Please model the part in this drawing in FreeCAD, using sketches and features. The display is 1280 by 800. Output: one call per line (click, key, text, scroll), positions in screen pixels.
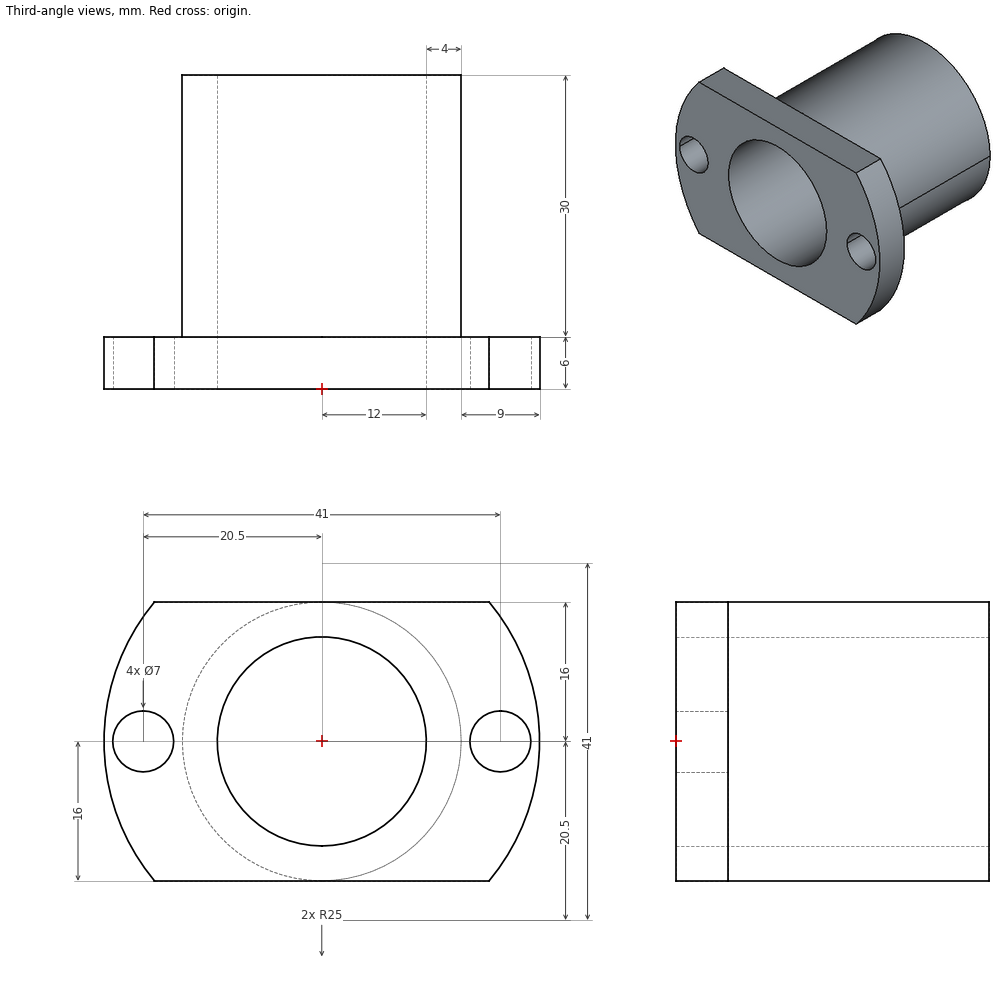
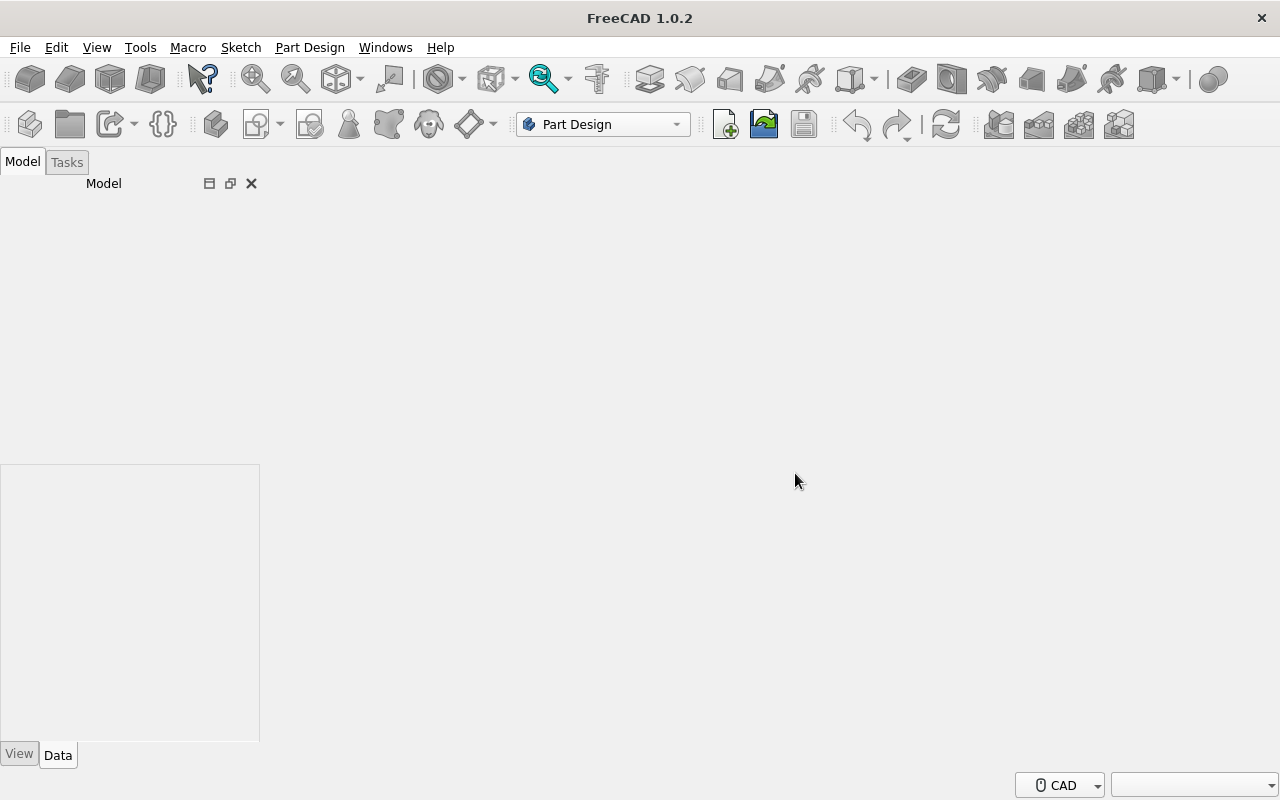
click(724, 124)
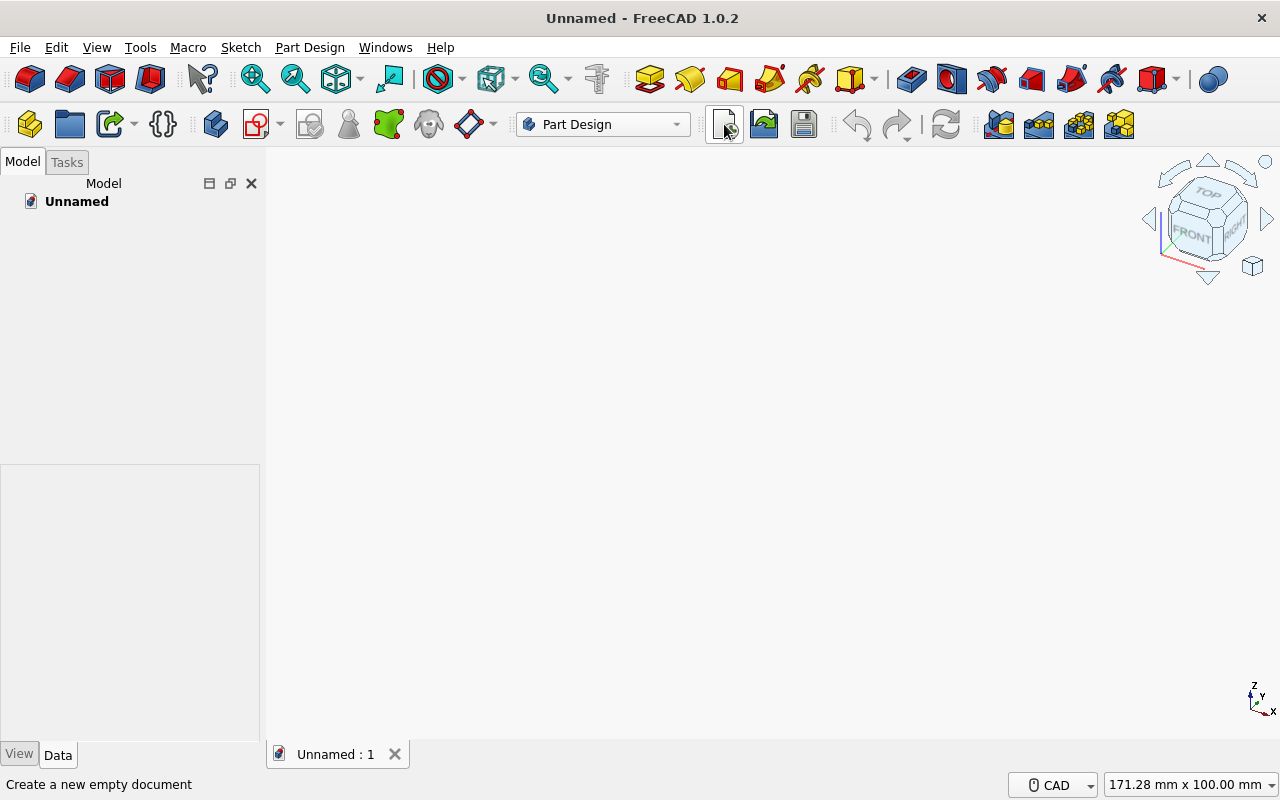
click(256, 124)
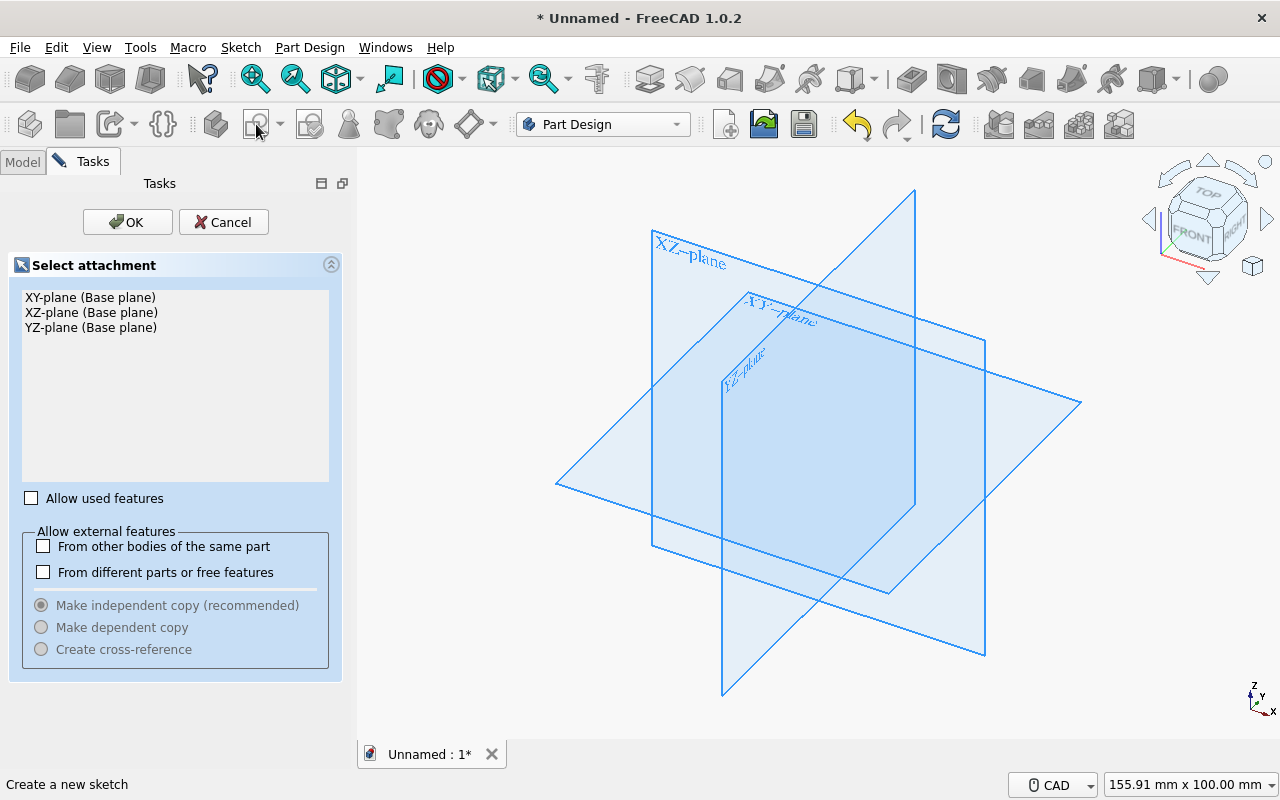
click(82, 298)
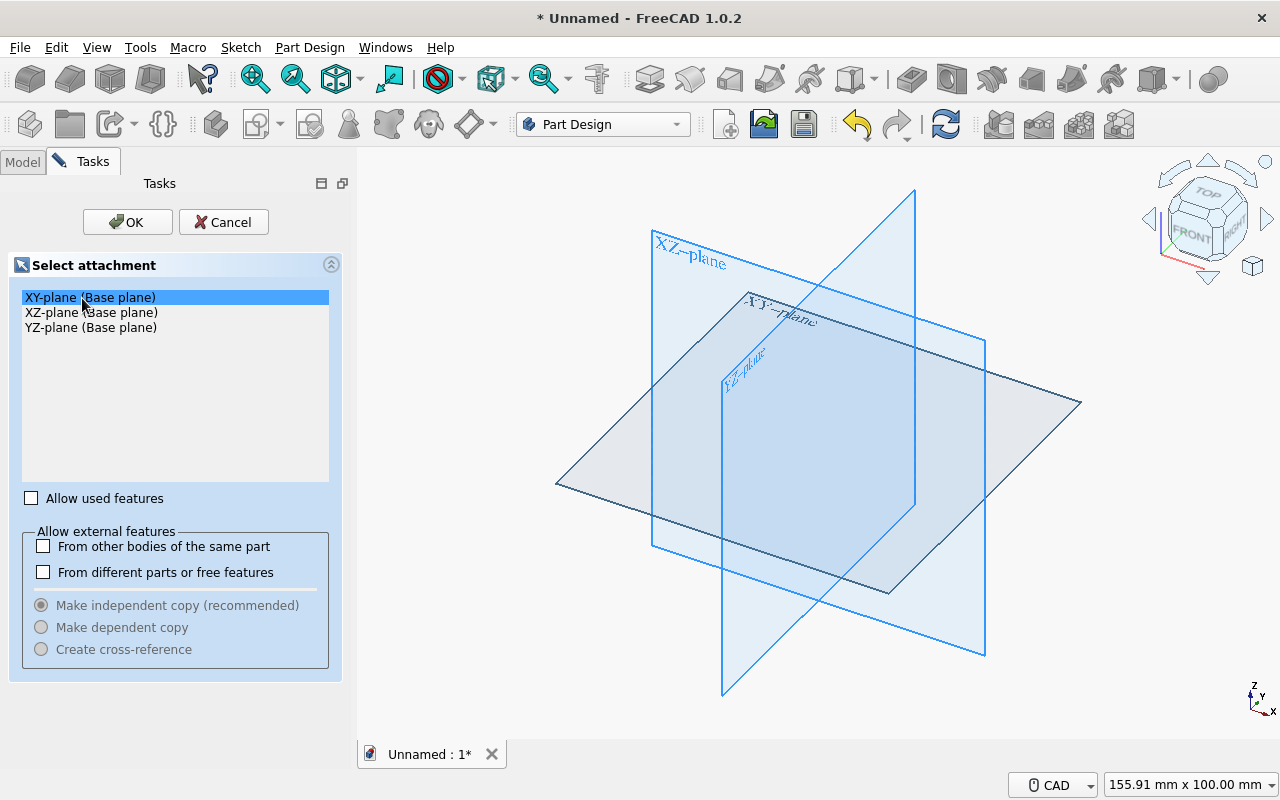
click(128, 222)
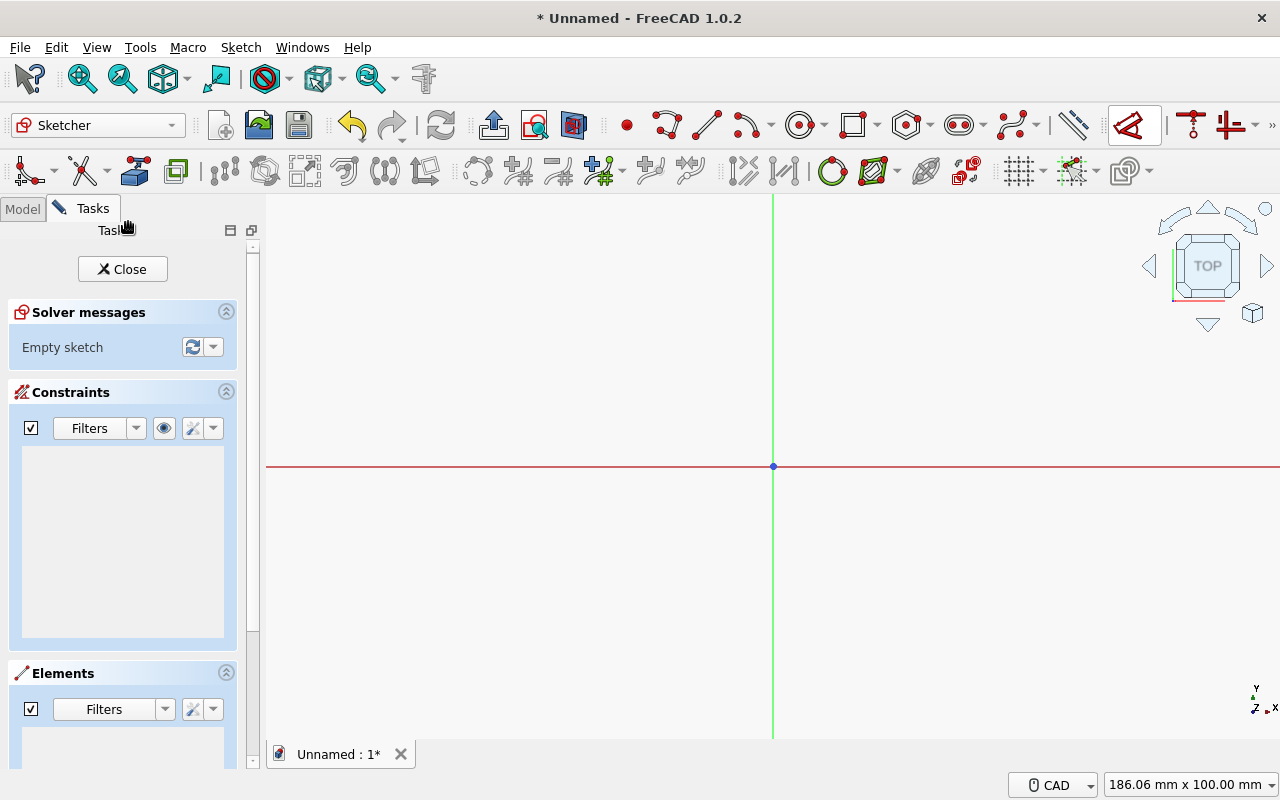
scroll(1007, 249, up, 3)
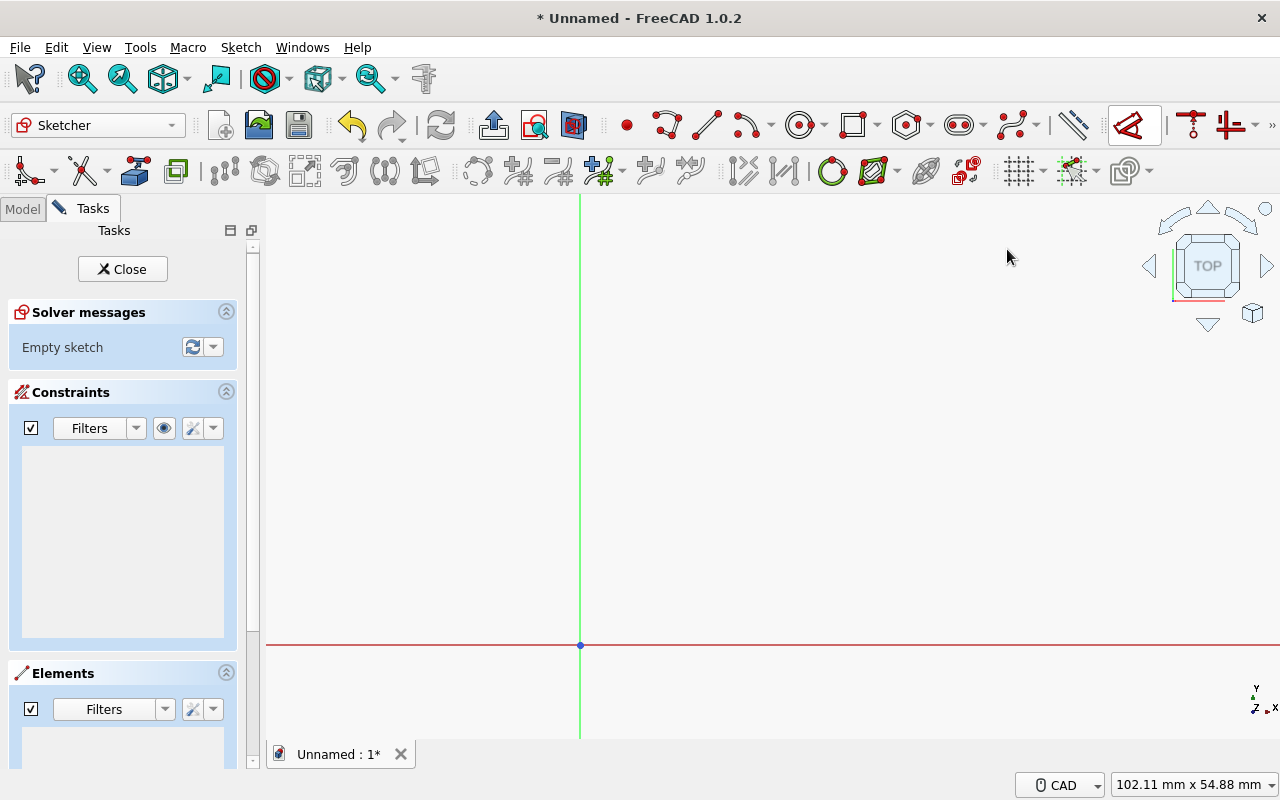
click(668, 126)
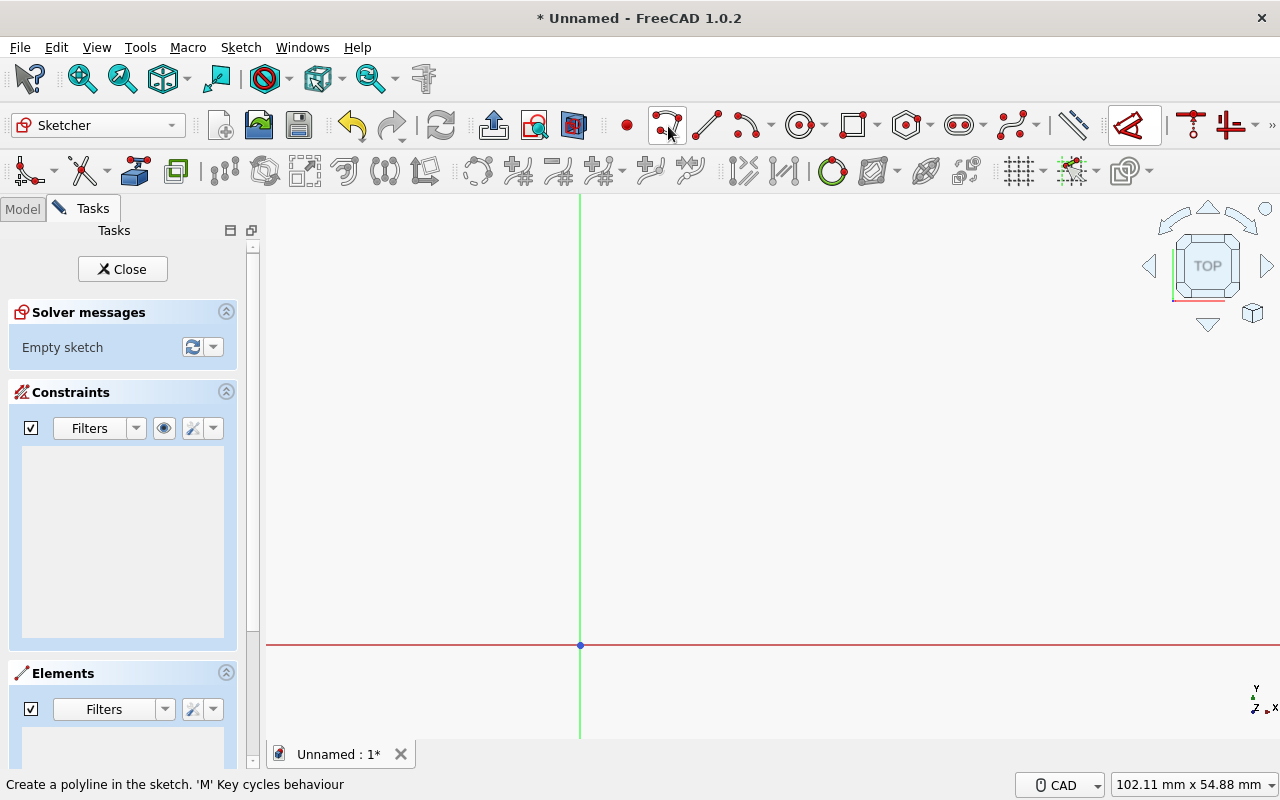
click(699, 645)
click(828, 636)
click(828, 586)
click(739, 586)
click(739, 288)
click(699, 288)
click(699, 645)
key(Escape)
key(Escape)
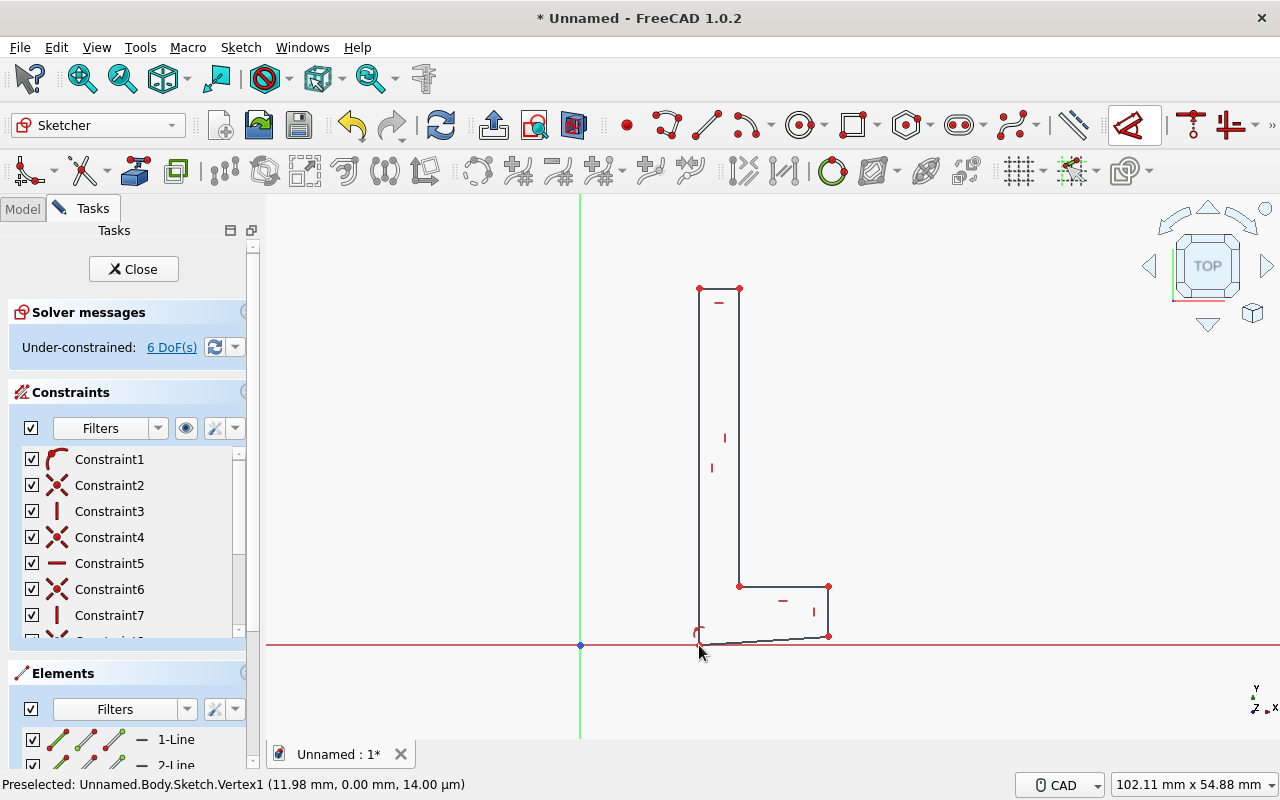
click(738, 643)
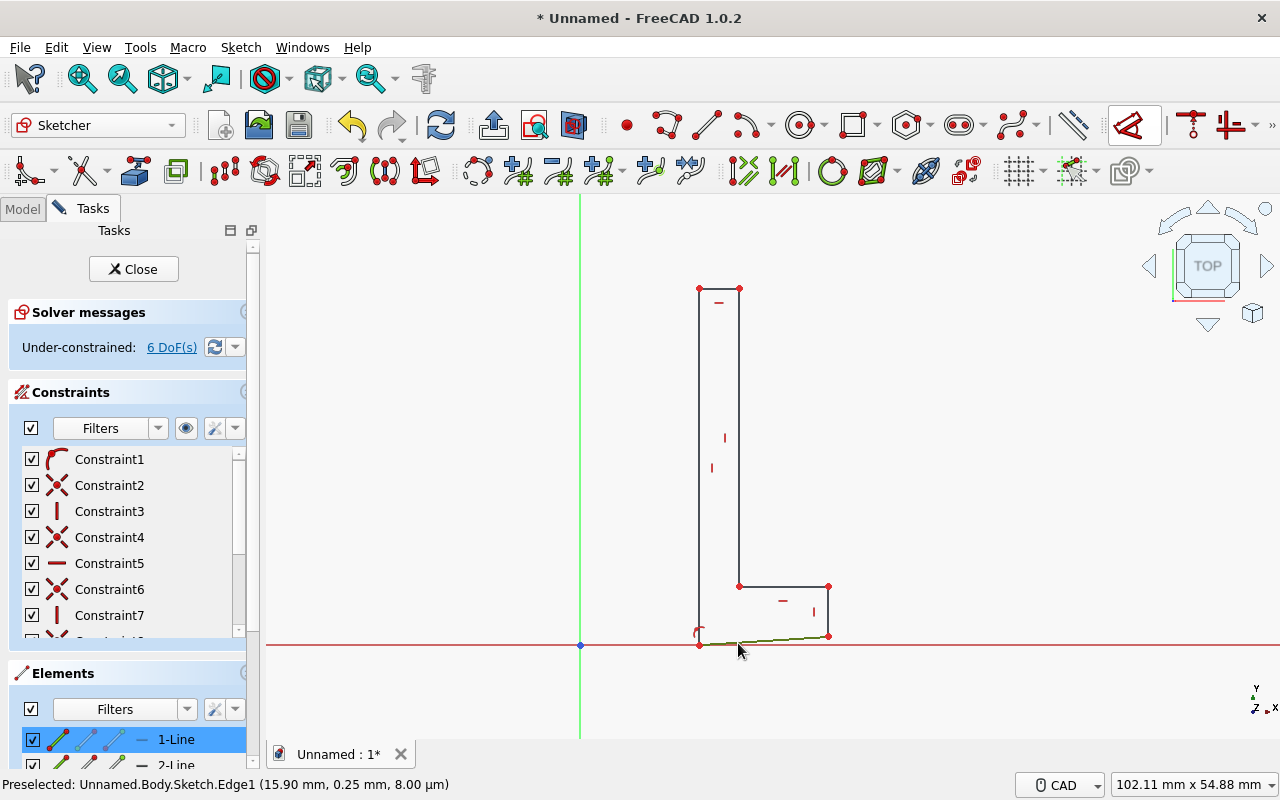
click(1258, 126)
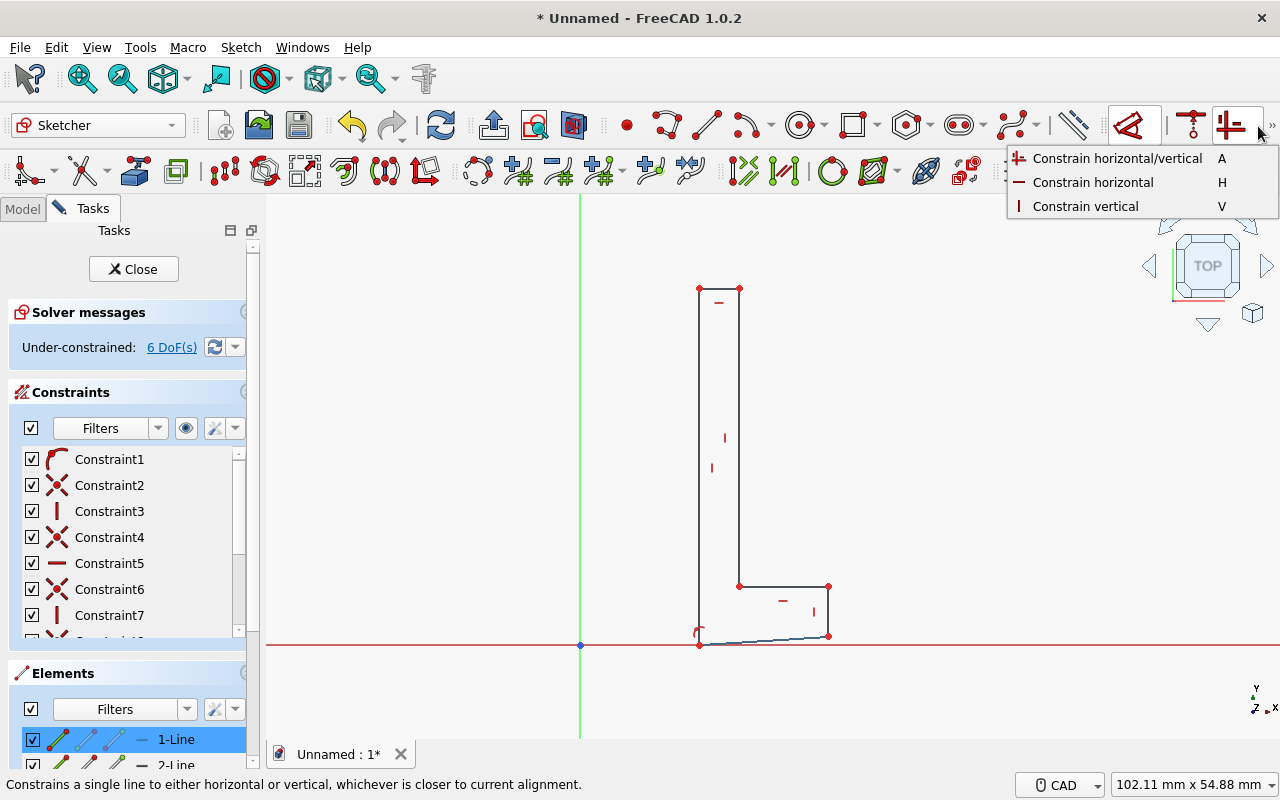
click(1143, 182)